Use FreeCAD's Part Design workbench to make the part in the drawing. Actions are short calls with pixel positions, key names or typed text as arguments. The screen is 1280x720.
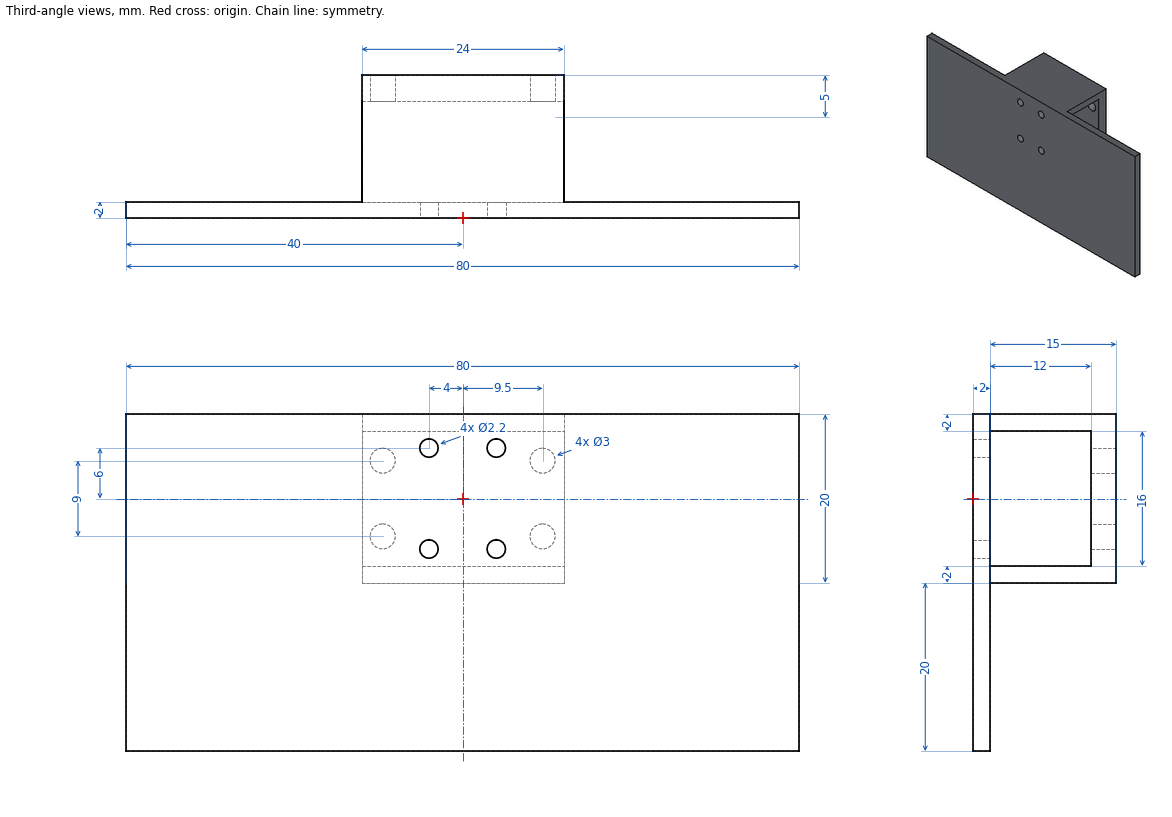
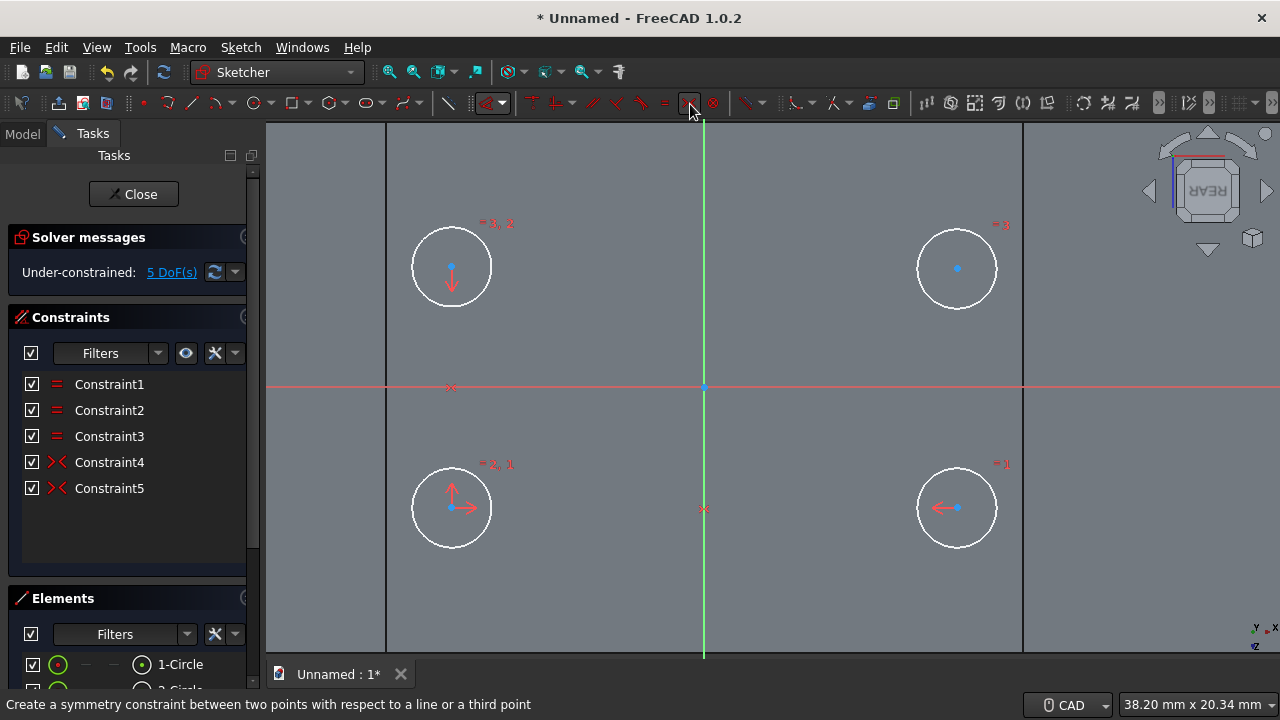
click(957, 508)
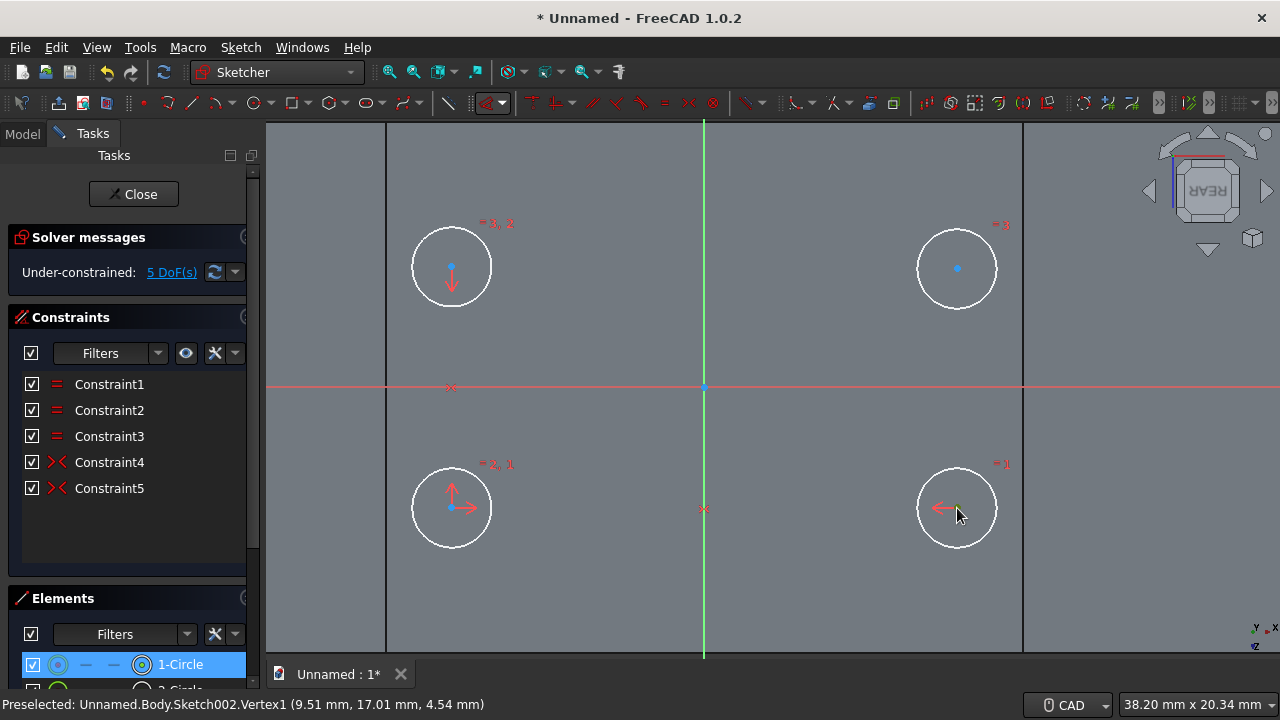
click(957, 269)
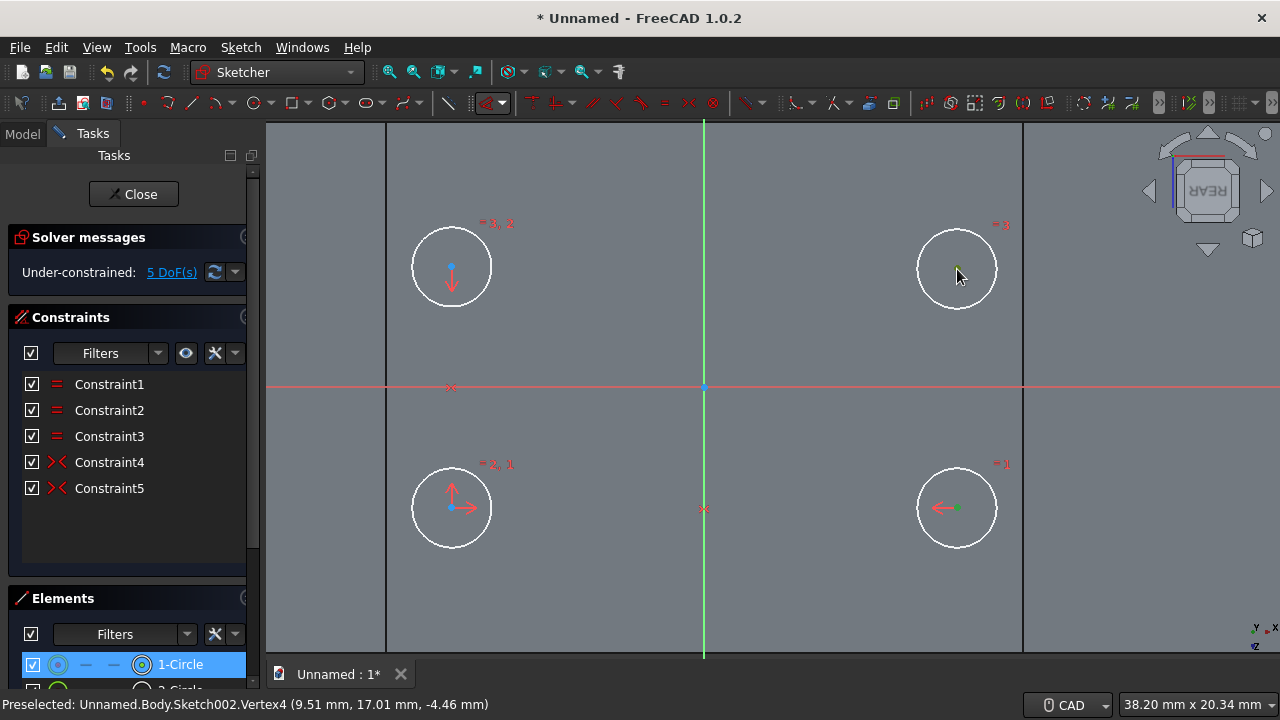
click(353, 387)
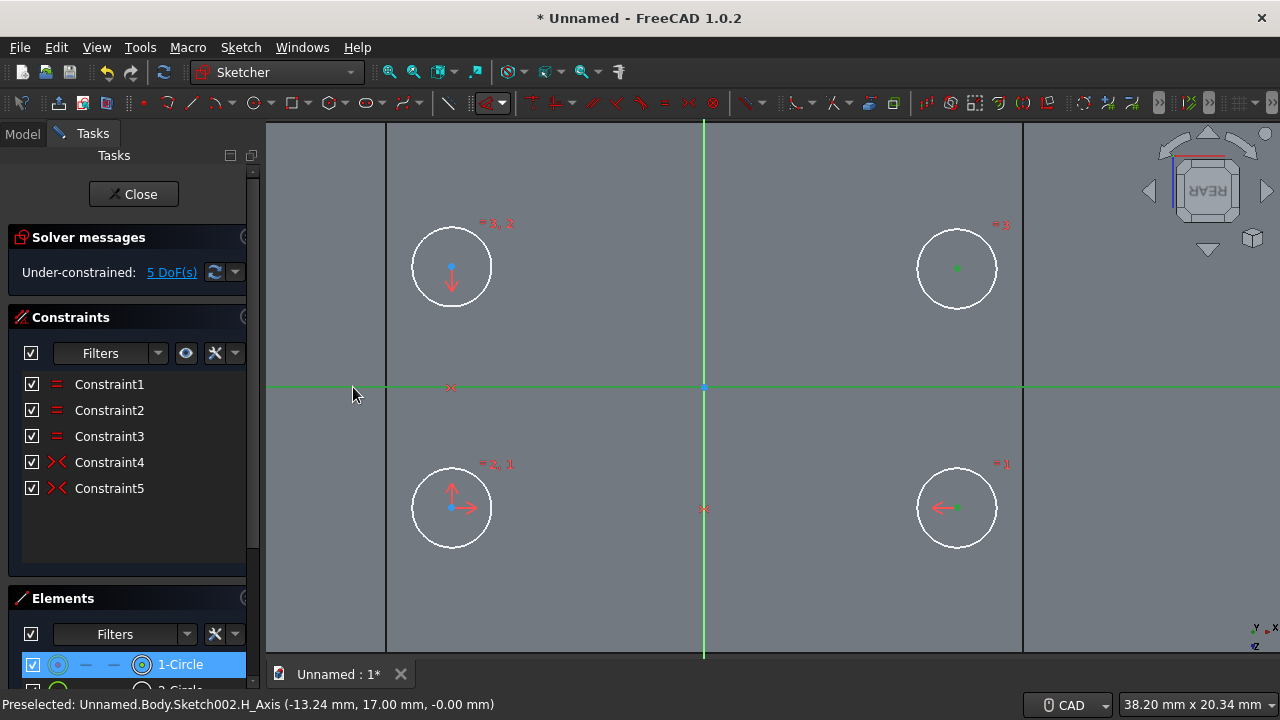
click(690, 104)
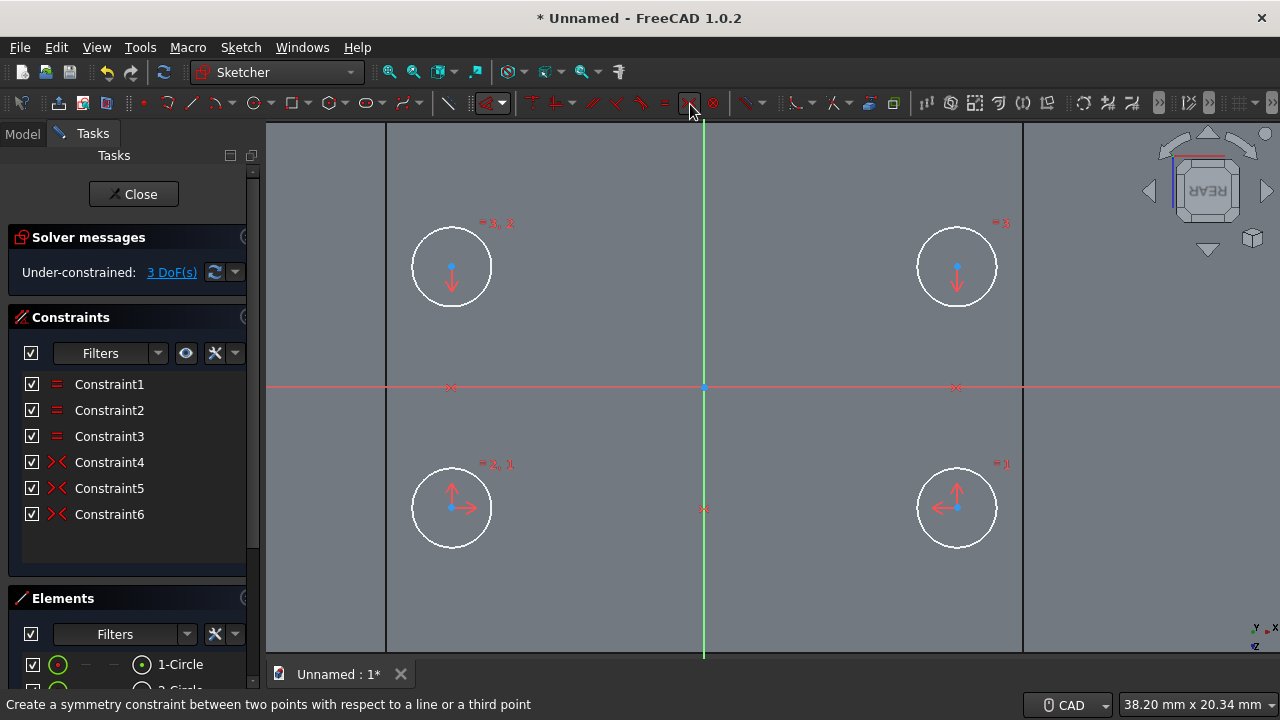
click(985, 480)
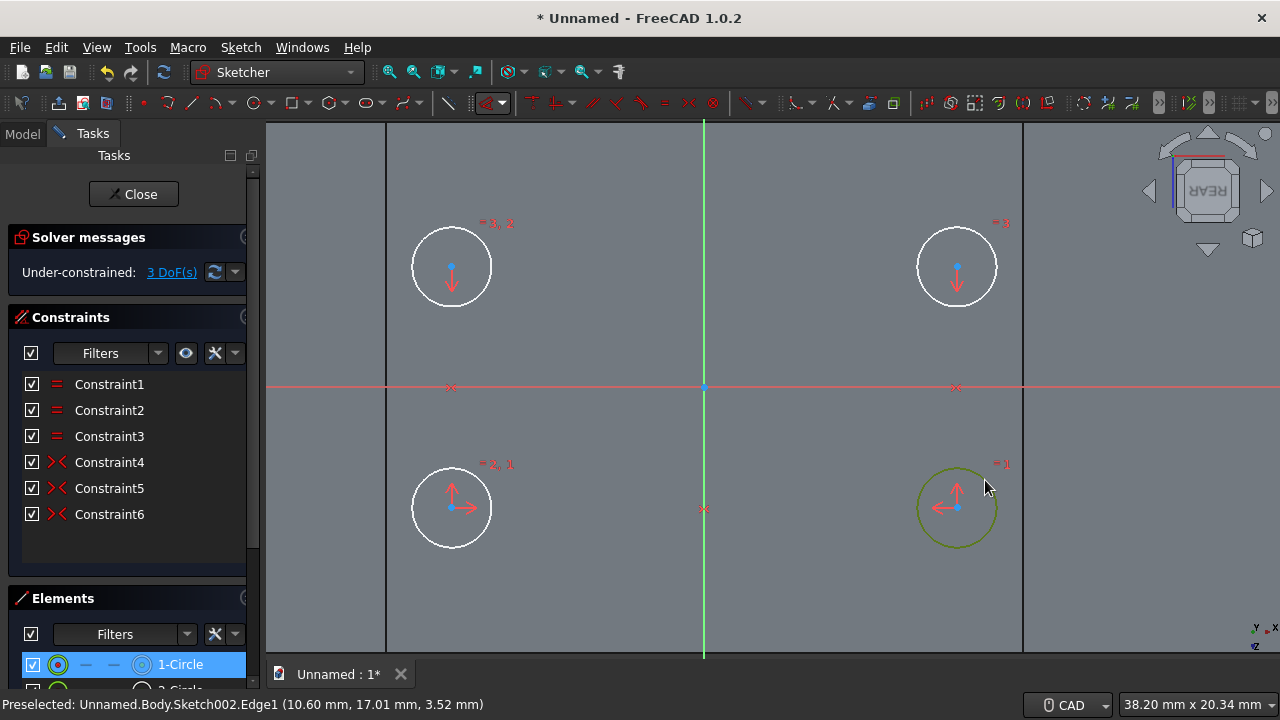
click(504, 104)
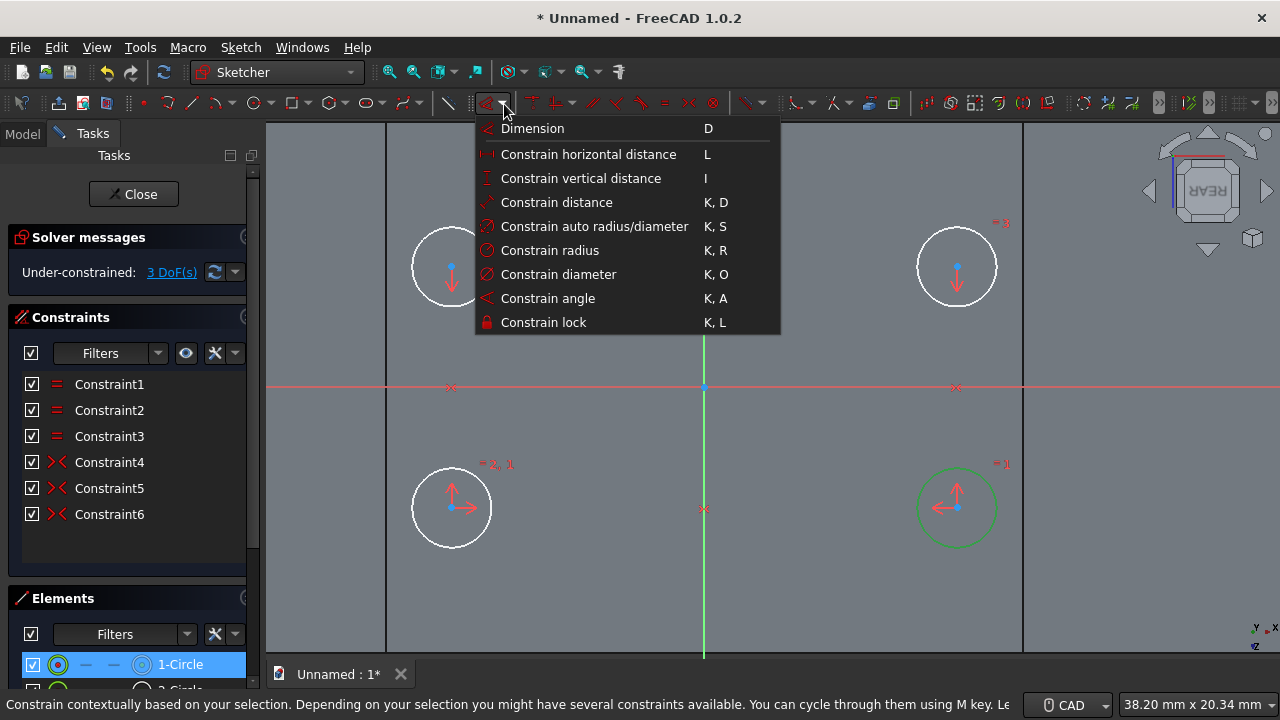
click(628, 274)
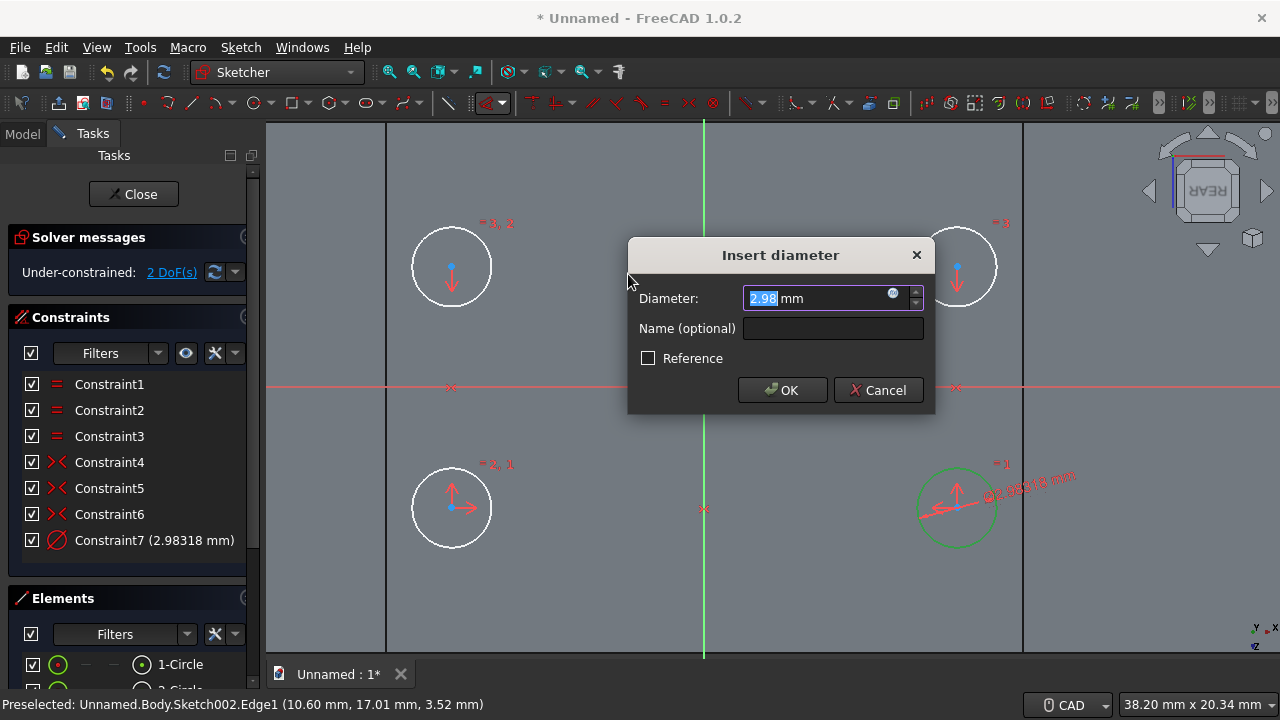
text(3)
key(Return)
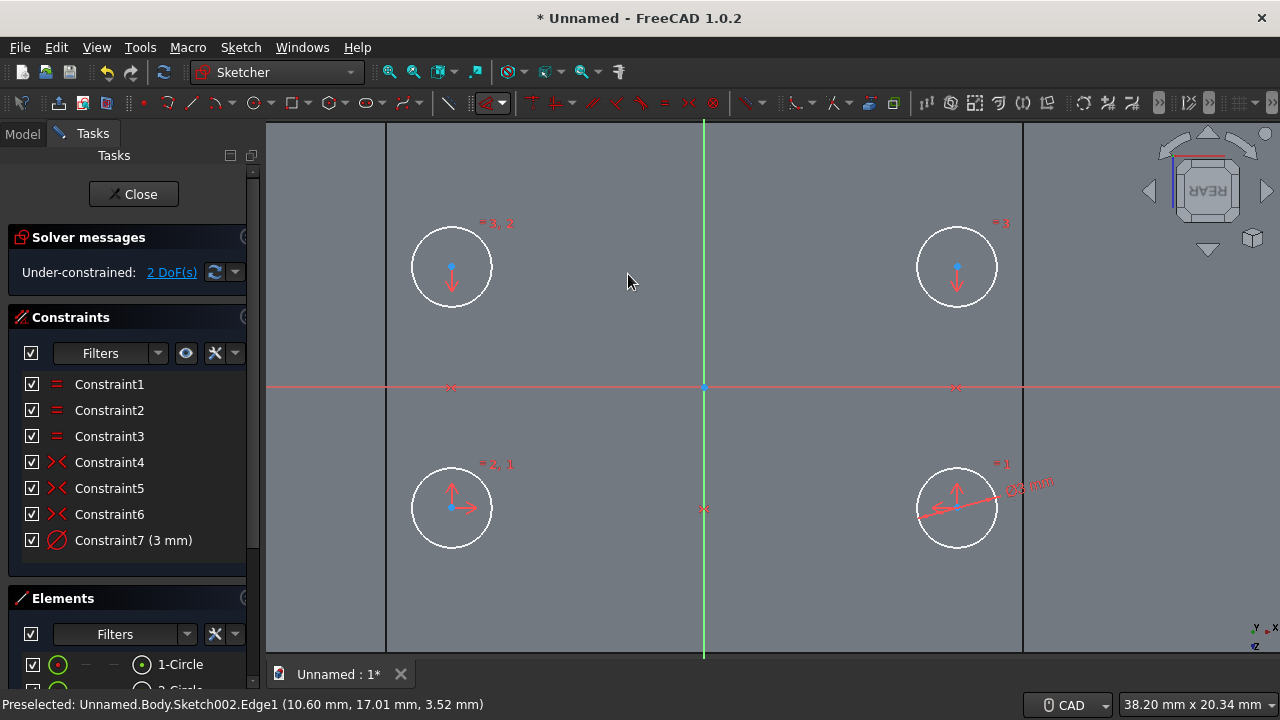
click(452, 508)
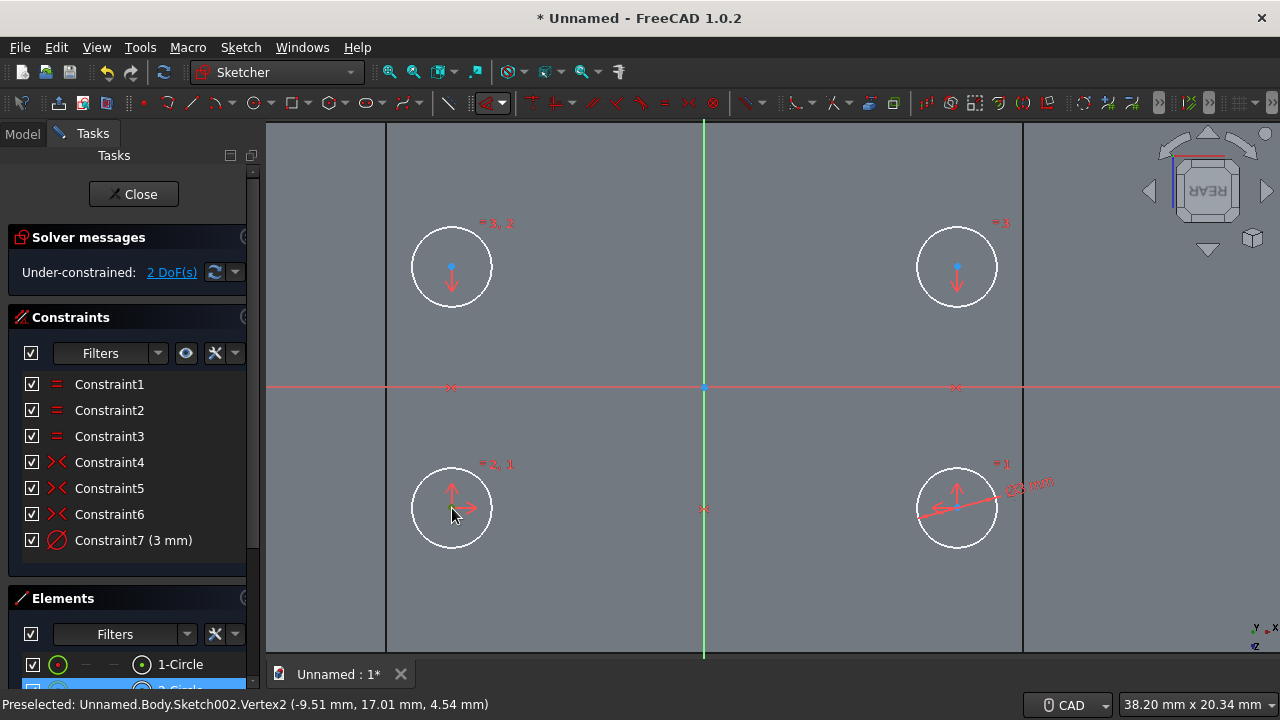
click(452, 267)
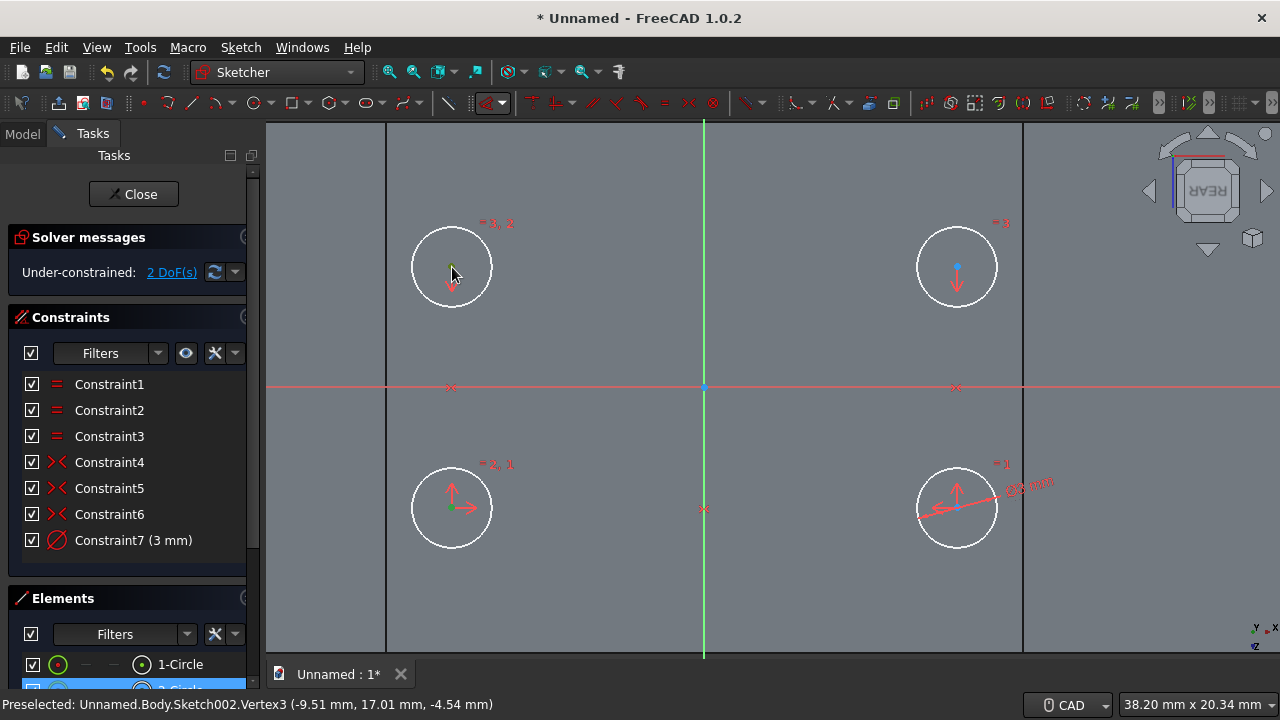
key(i)